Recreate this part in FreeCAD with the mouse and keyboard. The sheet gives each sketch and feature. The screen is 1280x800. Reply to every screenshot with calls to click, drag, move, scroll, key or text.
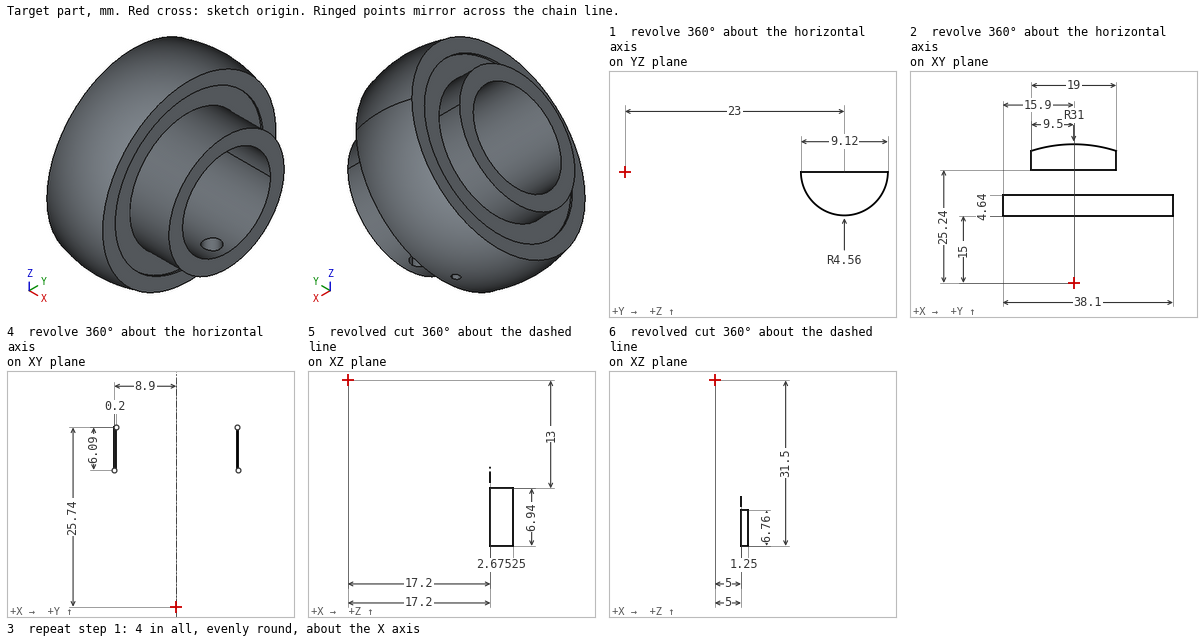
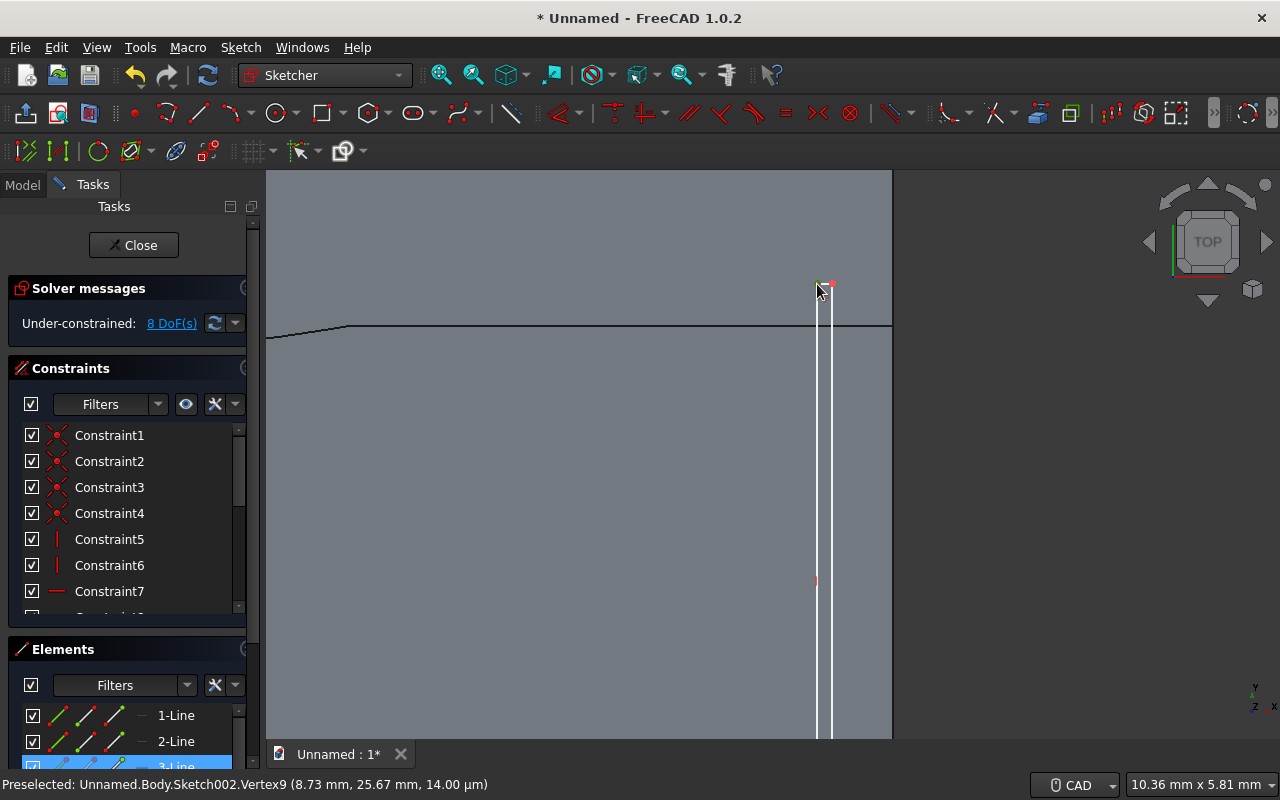
scroll(821, 285, down, 10)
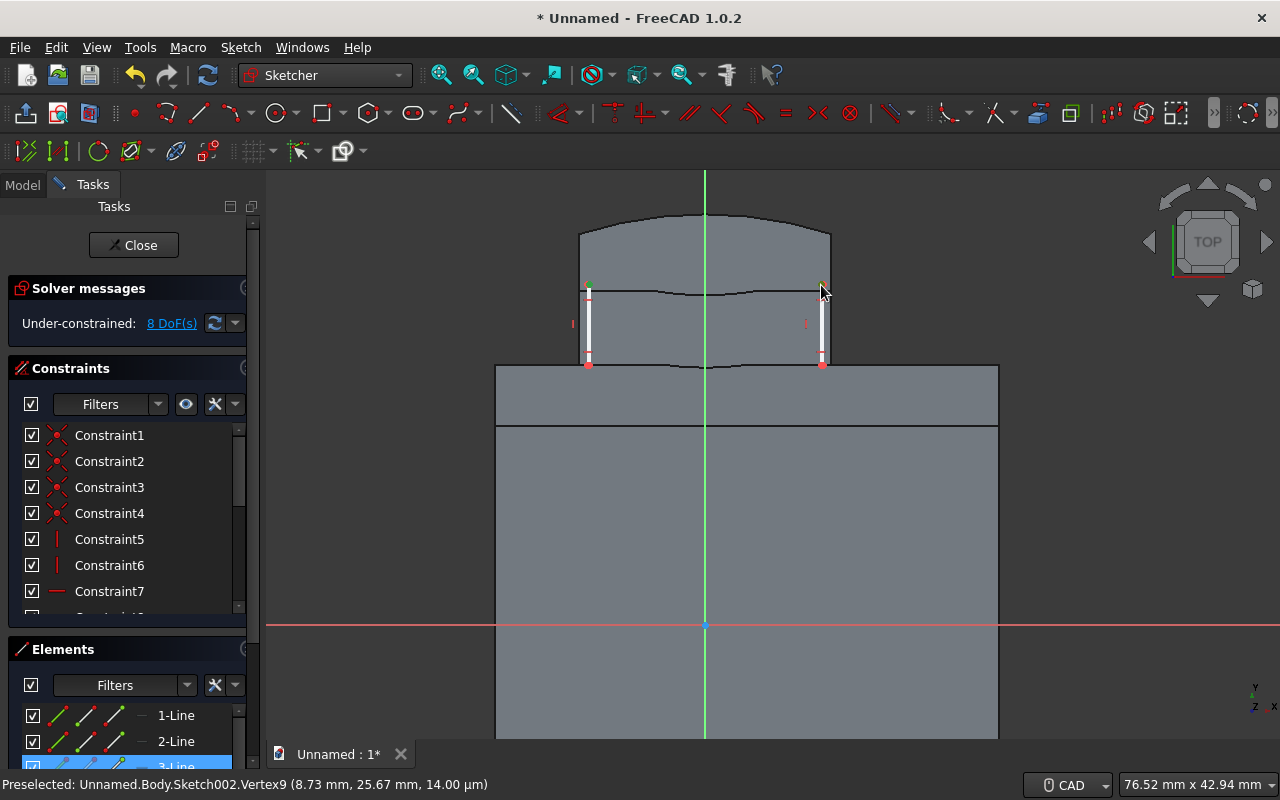
click(705, 674)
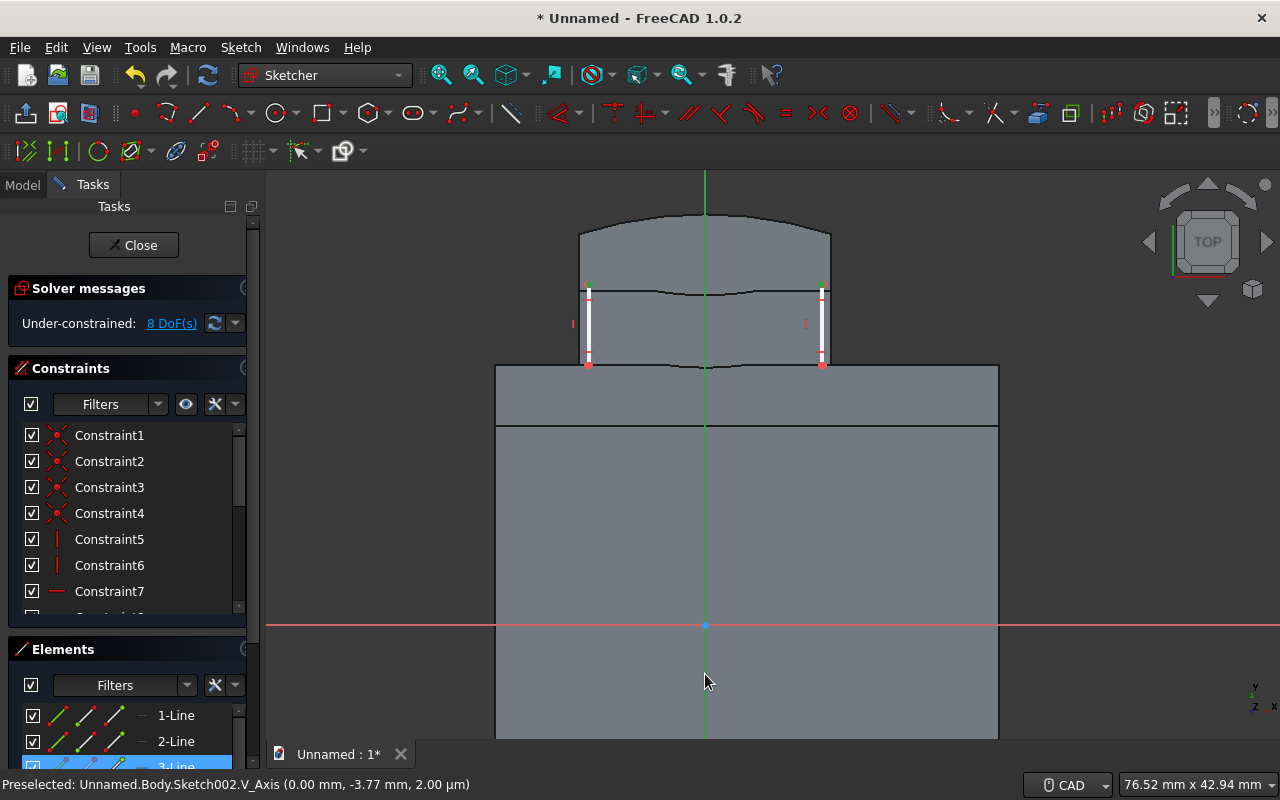
key(s)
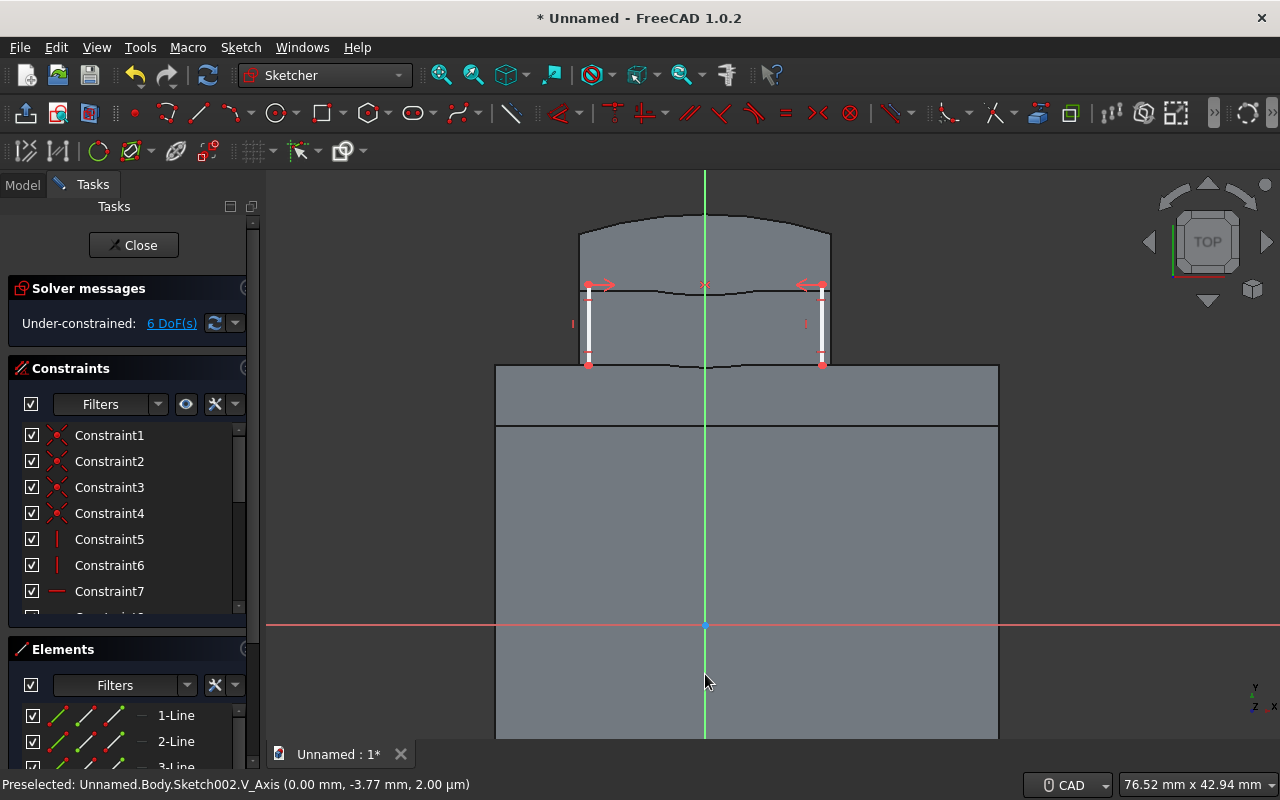
scroll(588, 366, up, 10)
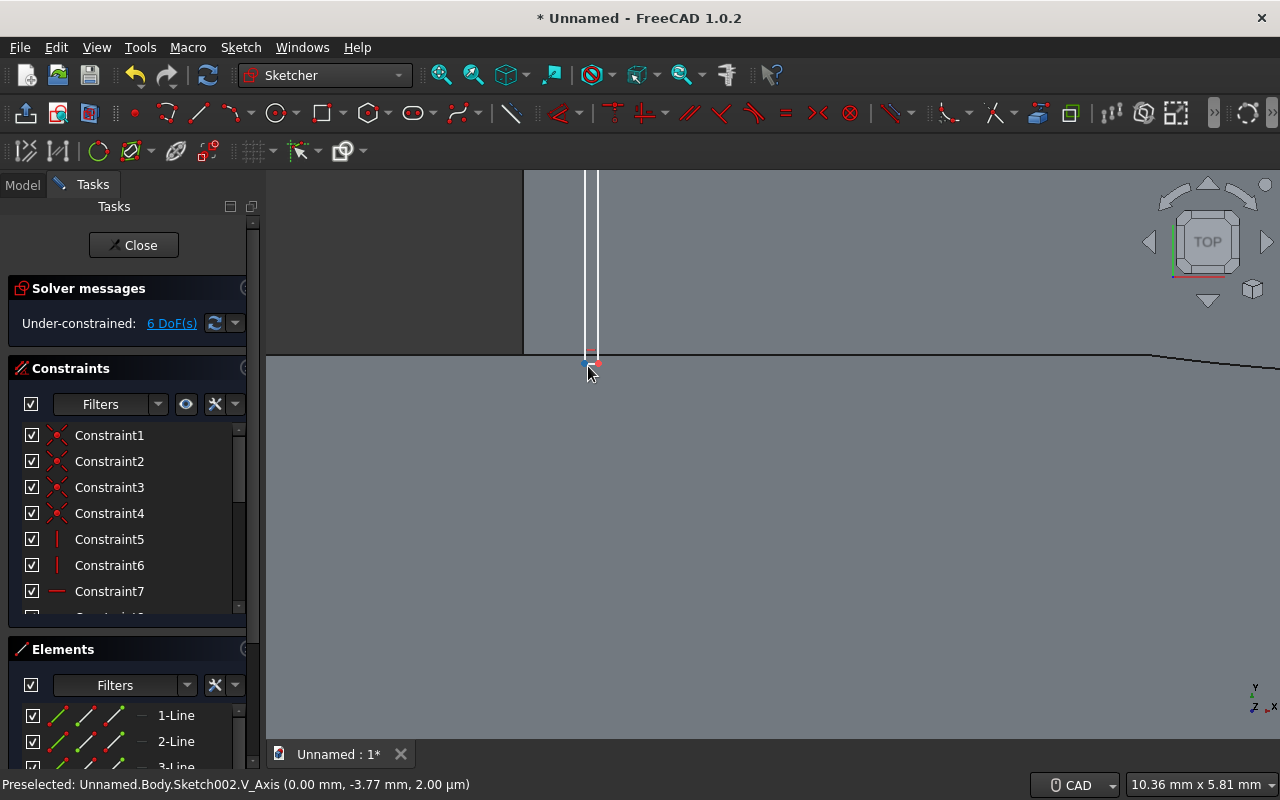
click(585, 364)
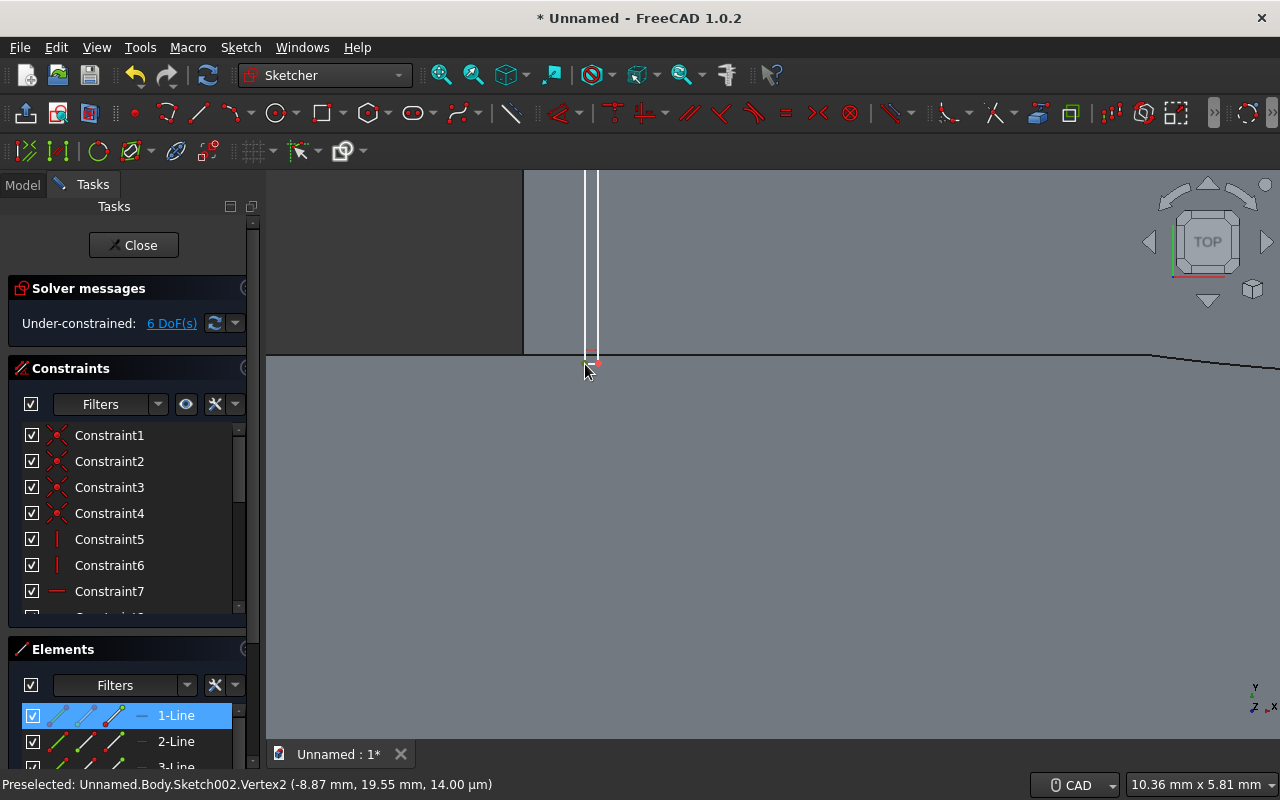
scroll(587, 366, down, 10)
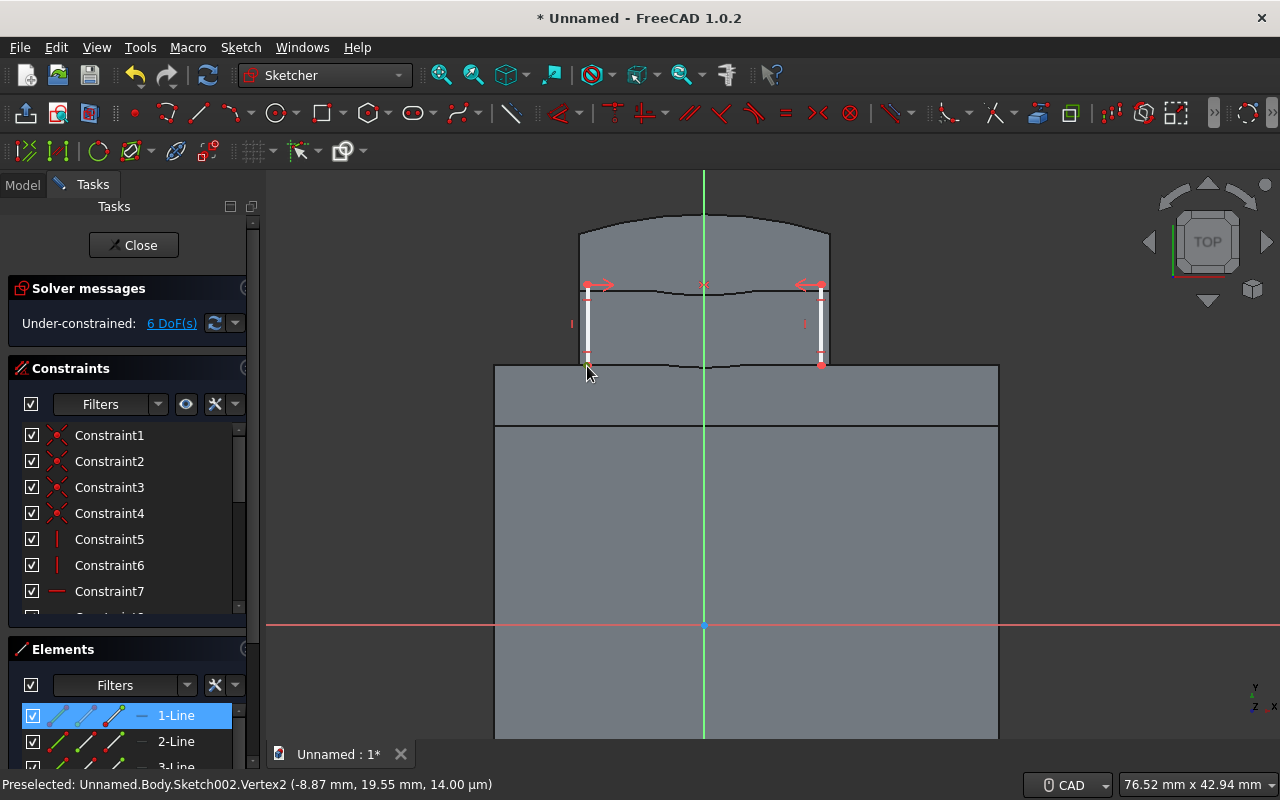
scroll(822, 366, up, 10)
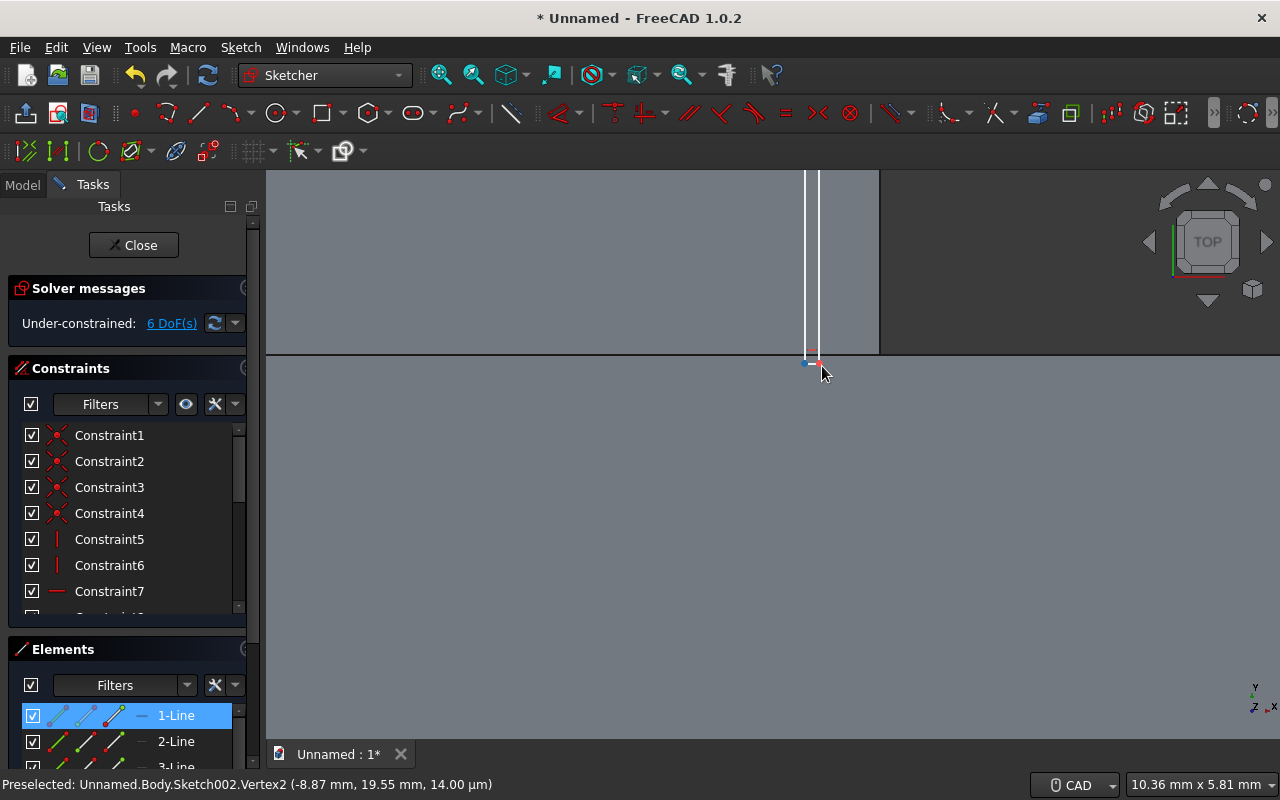
click(819, 364)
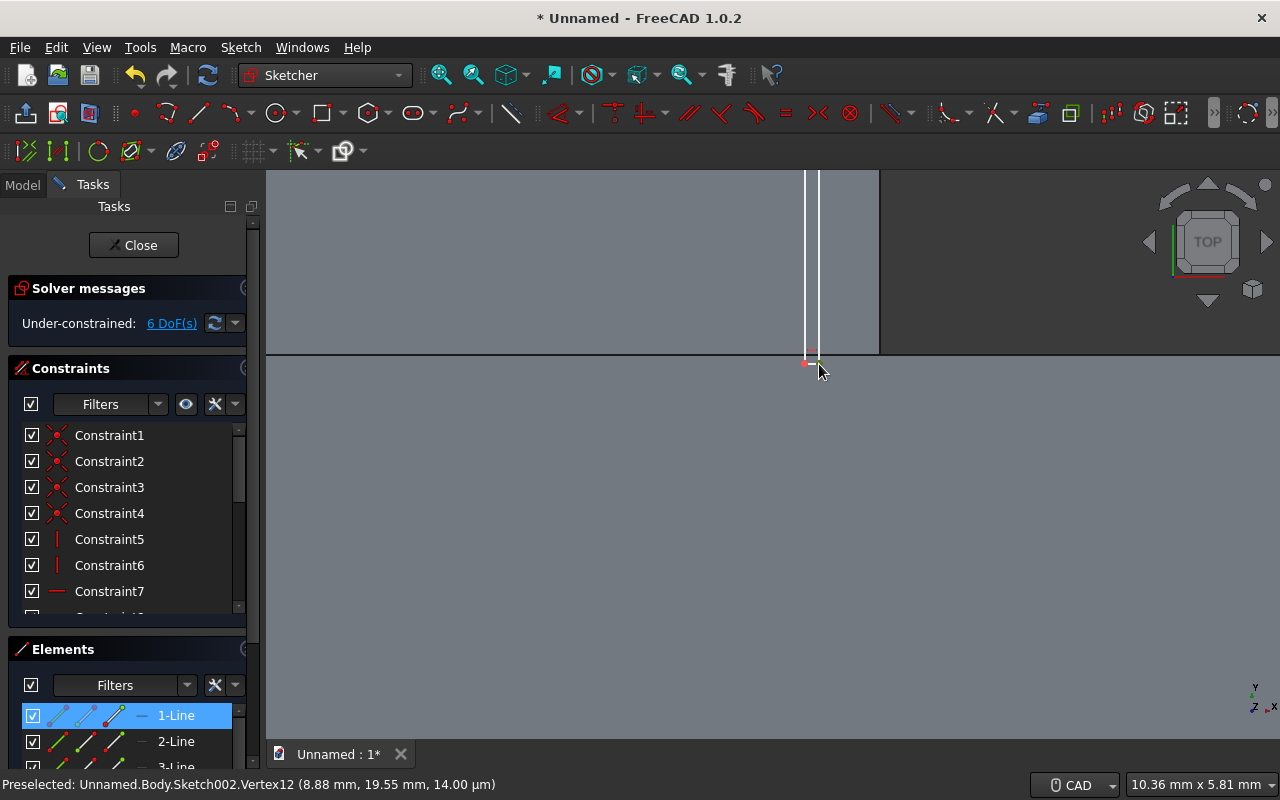
scroll(823, 366, down, 10)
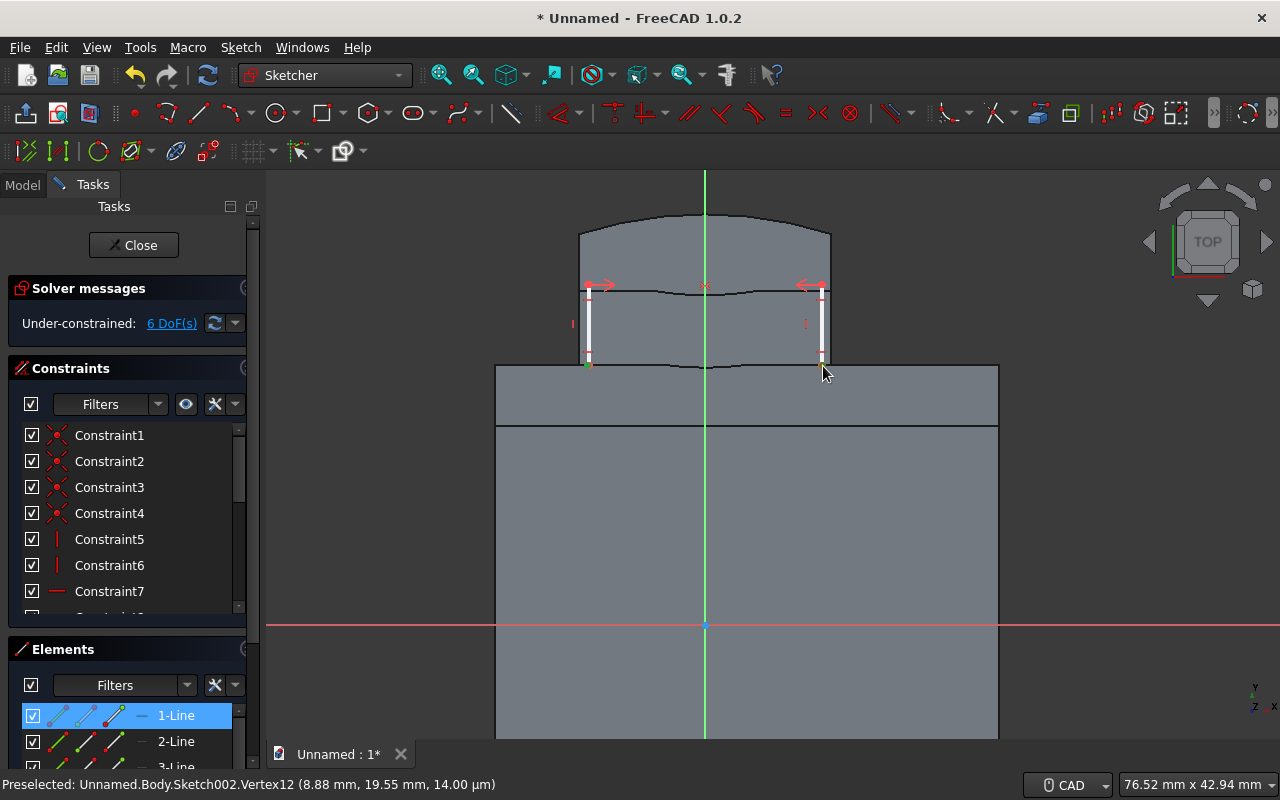
click(705, 674)